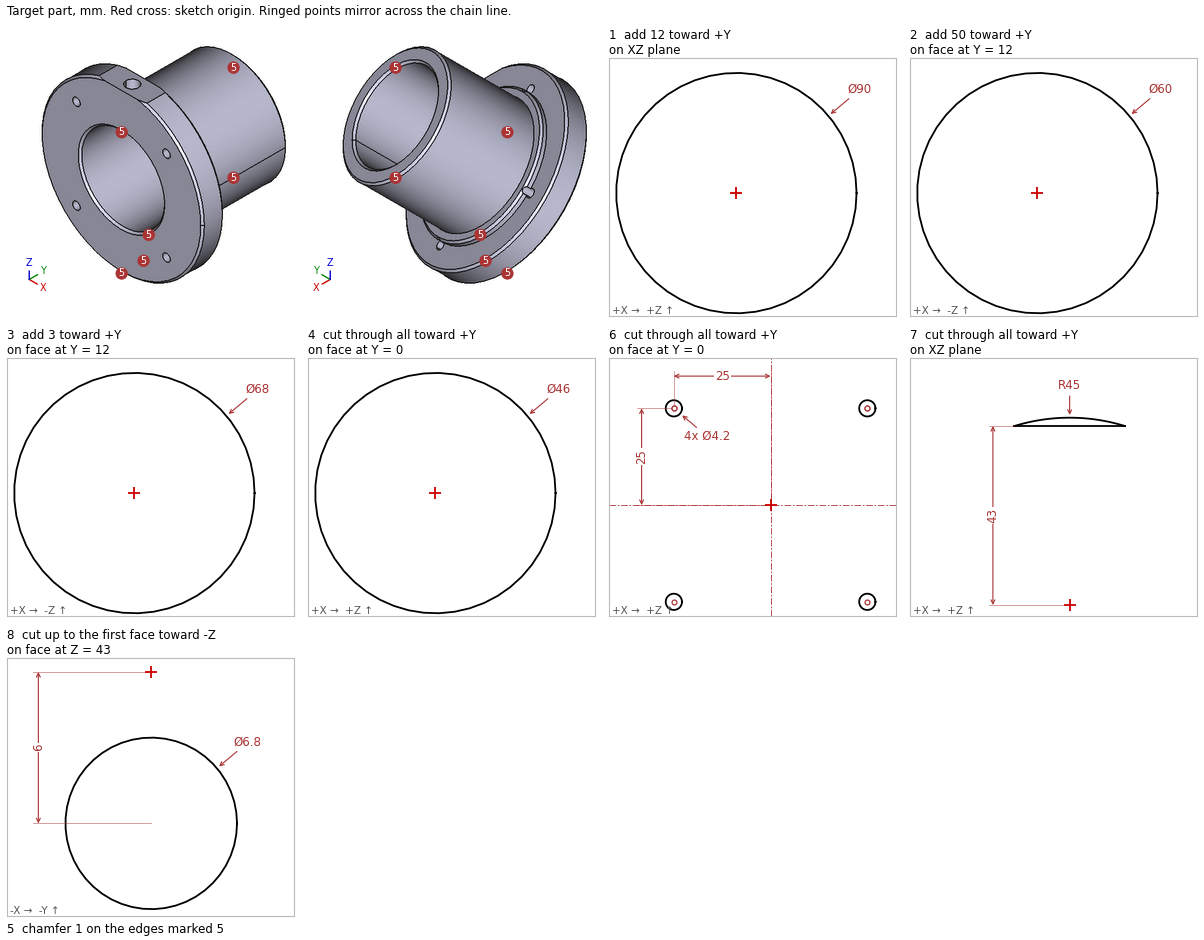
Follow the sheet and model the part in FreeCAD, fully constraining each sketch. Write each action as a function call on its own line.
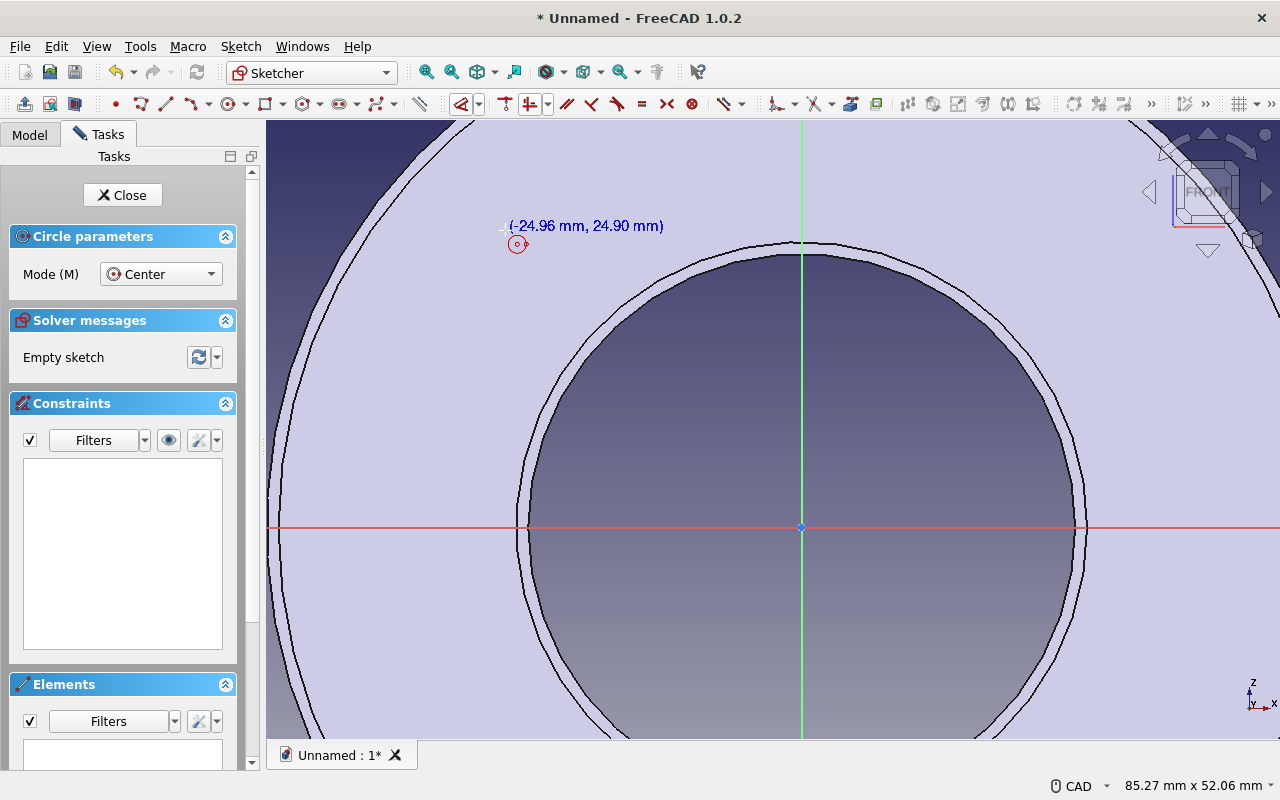
click(504, 230)
move(522, 213)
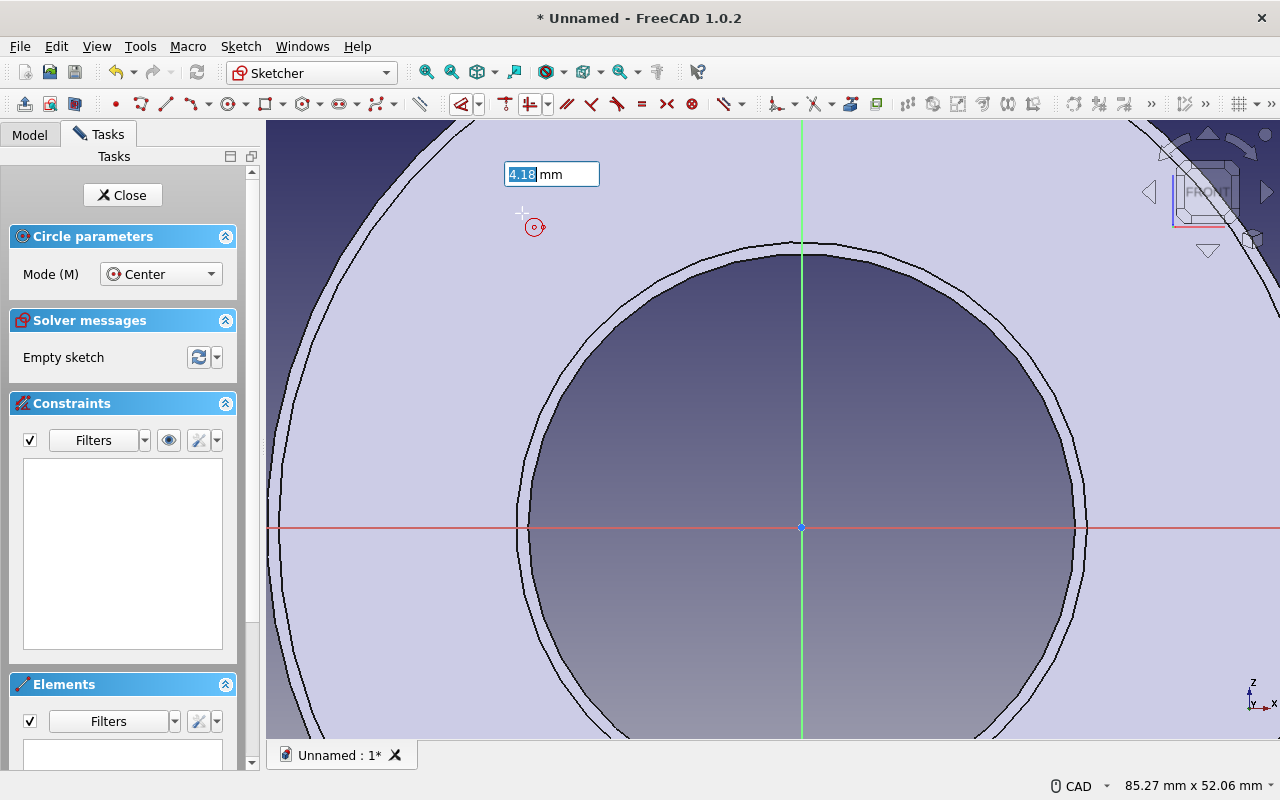
text(4.2)
key(Return)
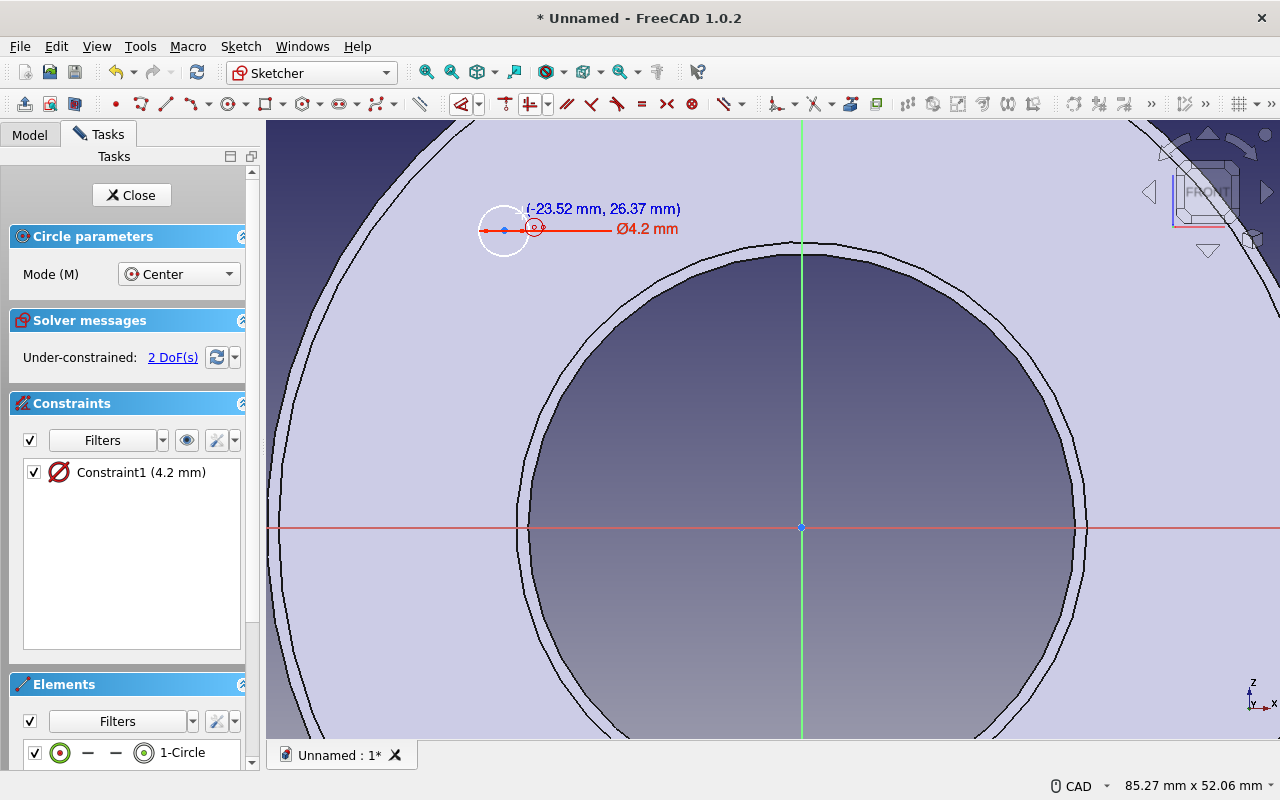
click(1099, 230)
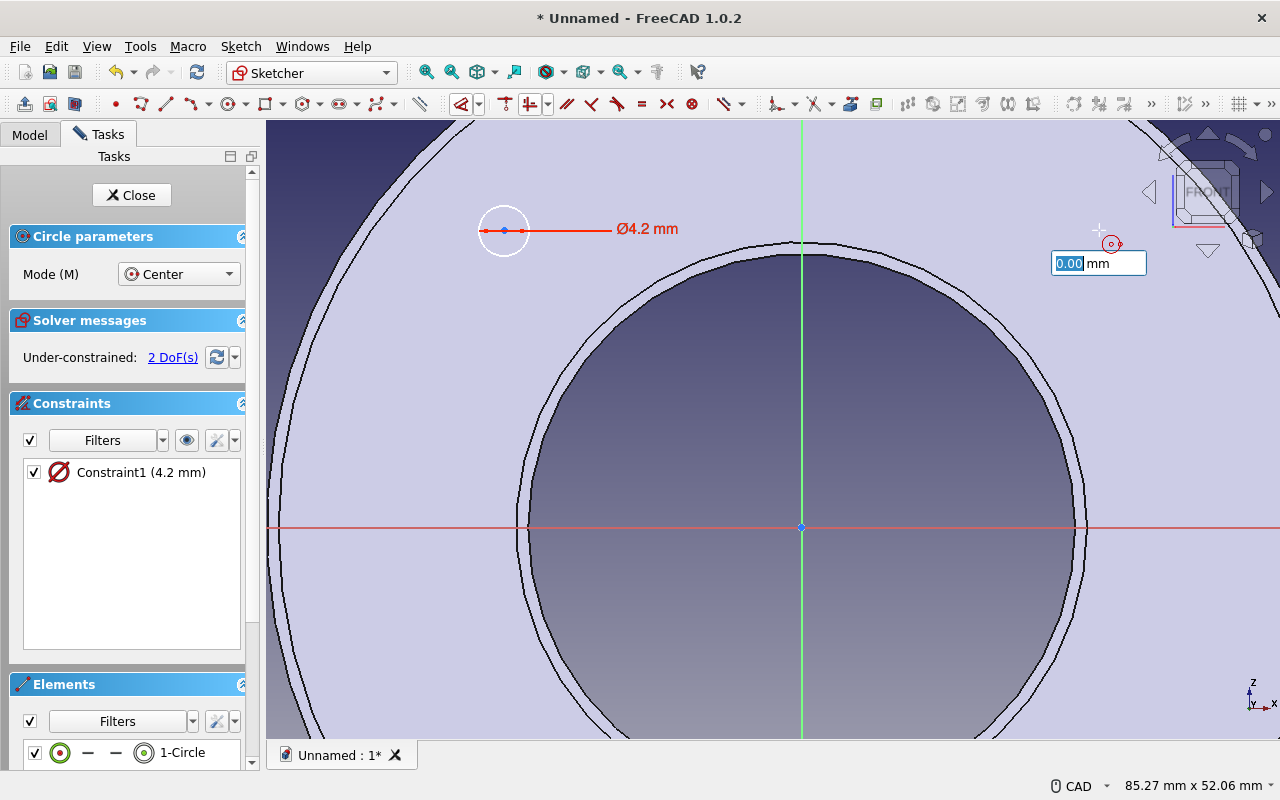
scroll(507, 230, down, 2)
move(916, 218)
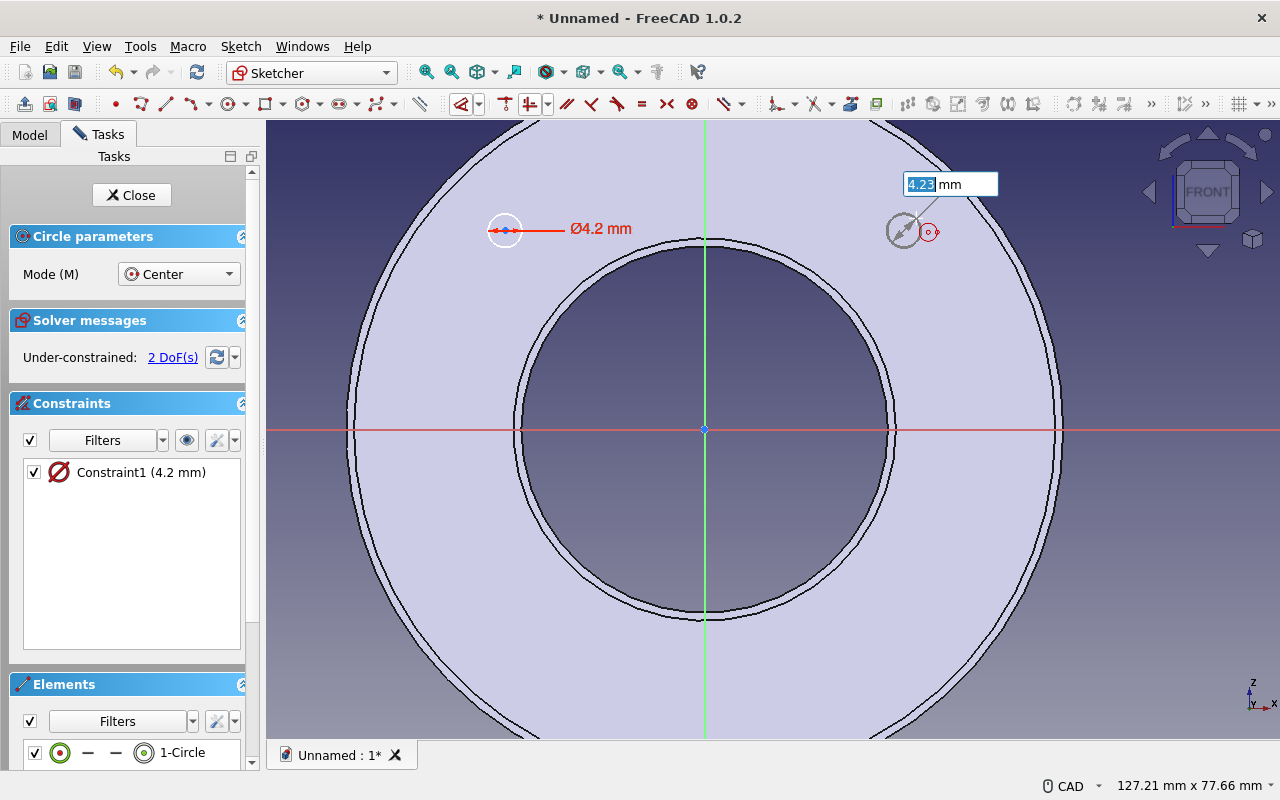
text(4.2)
key(Return)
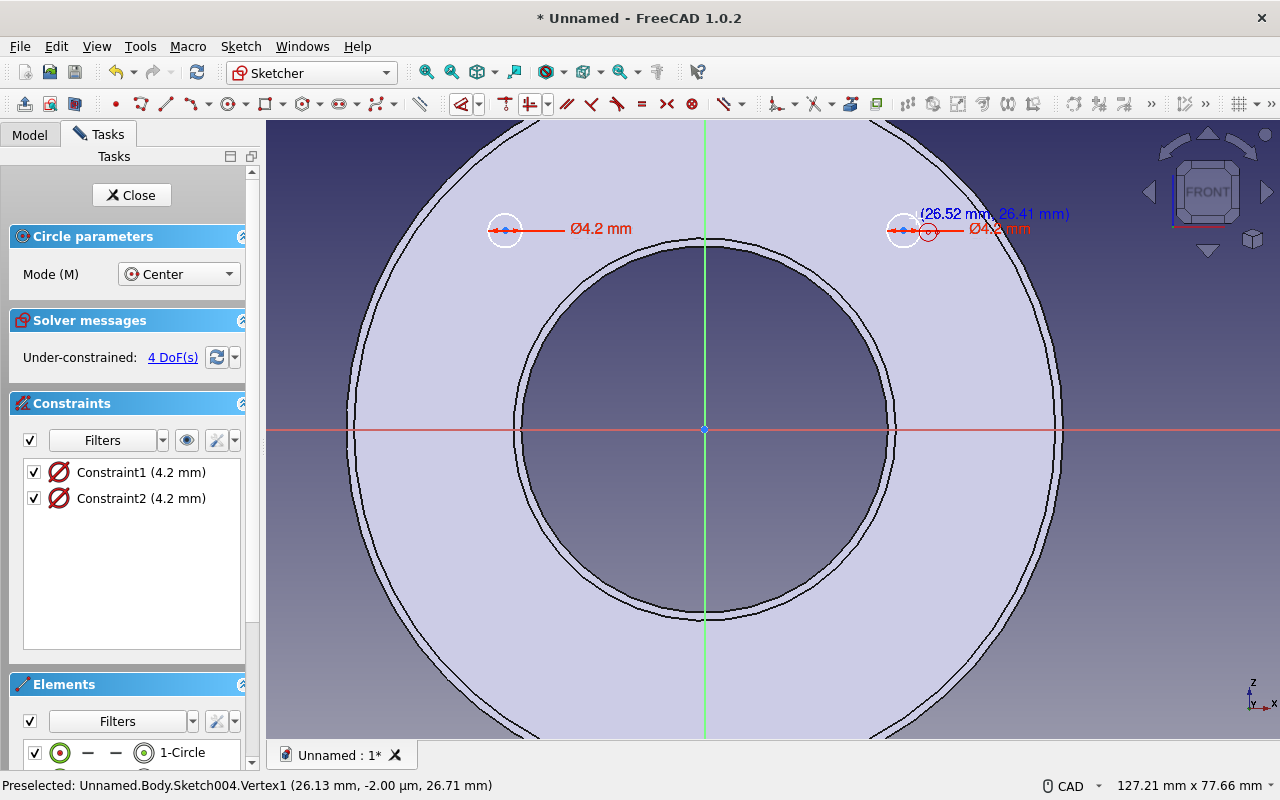
scroll(904, 629, up, 2)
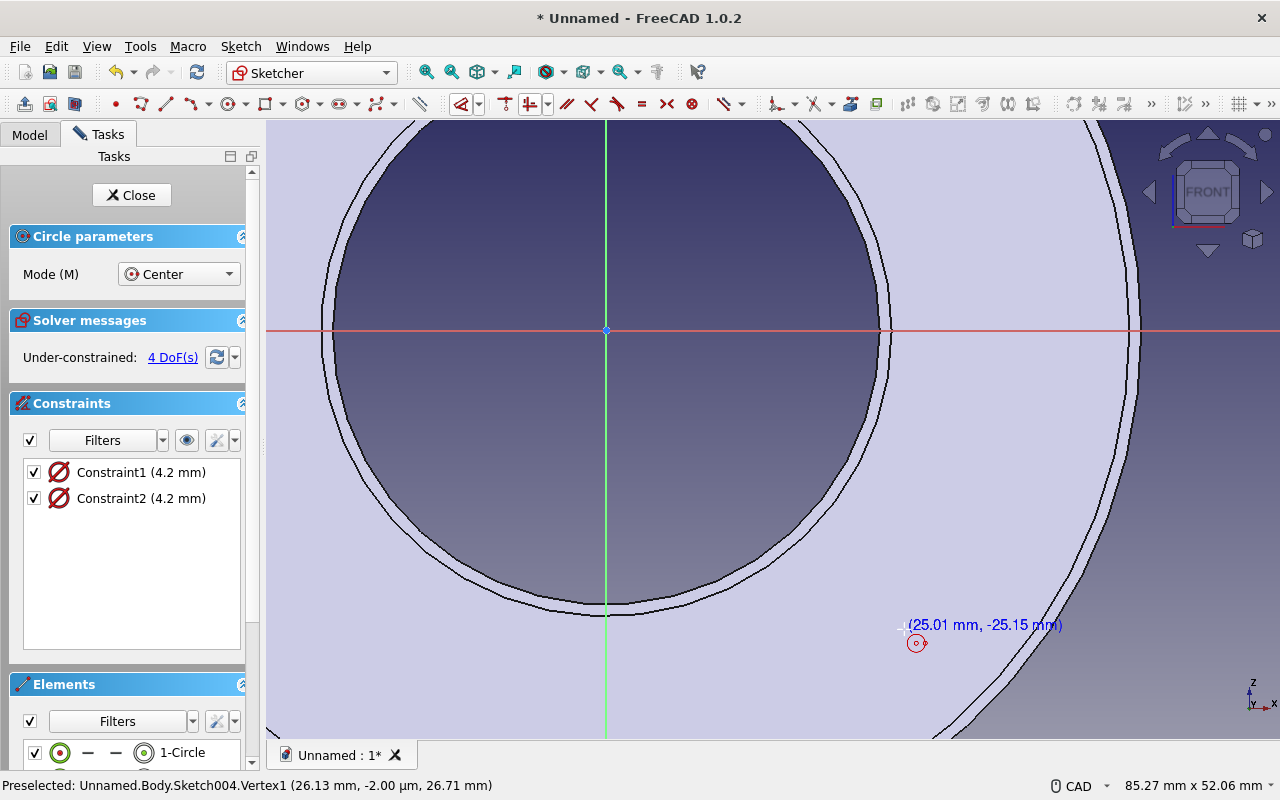
click(904, 628)
move(921, 611)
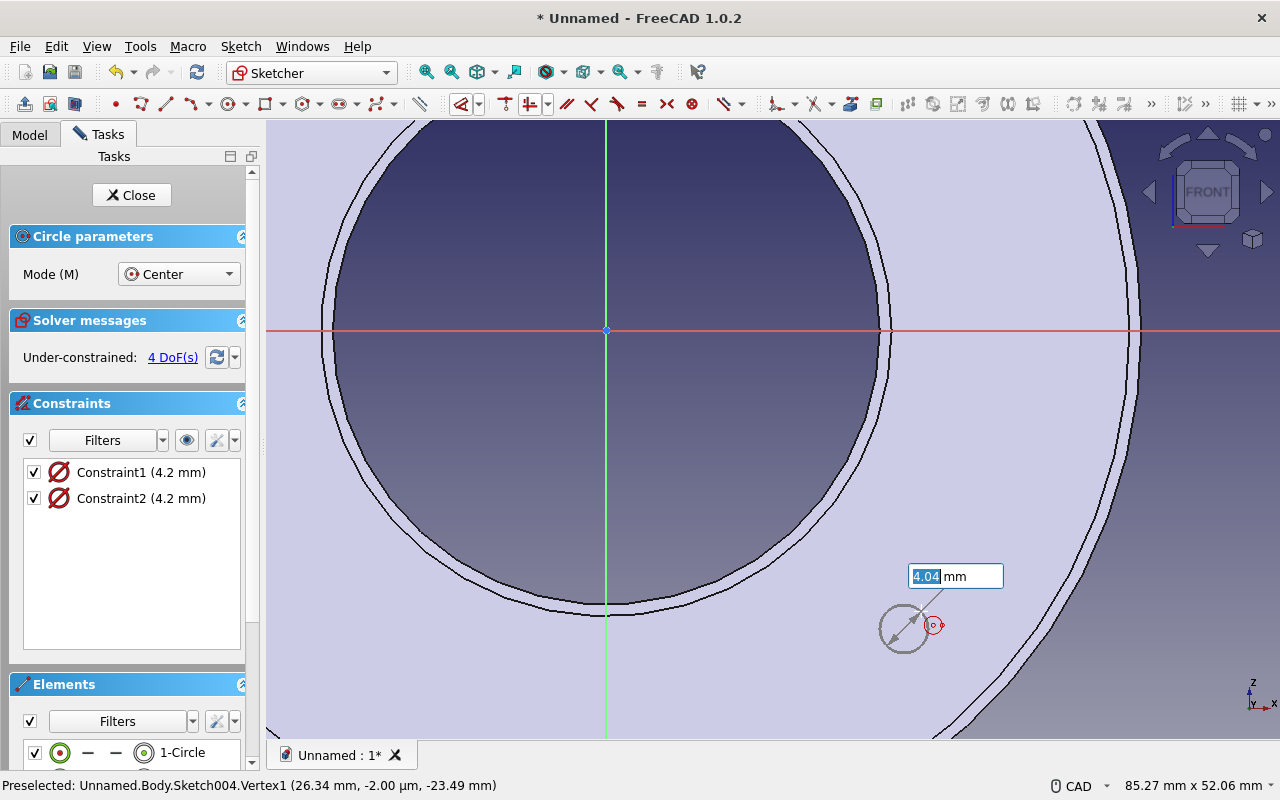
text(4.2)
key(Return)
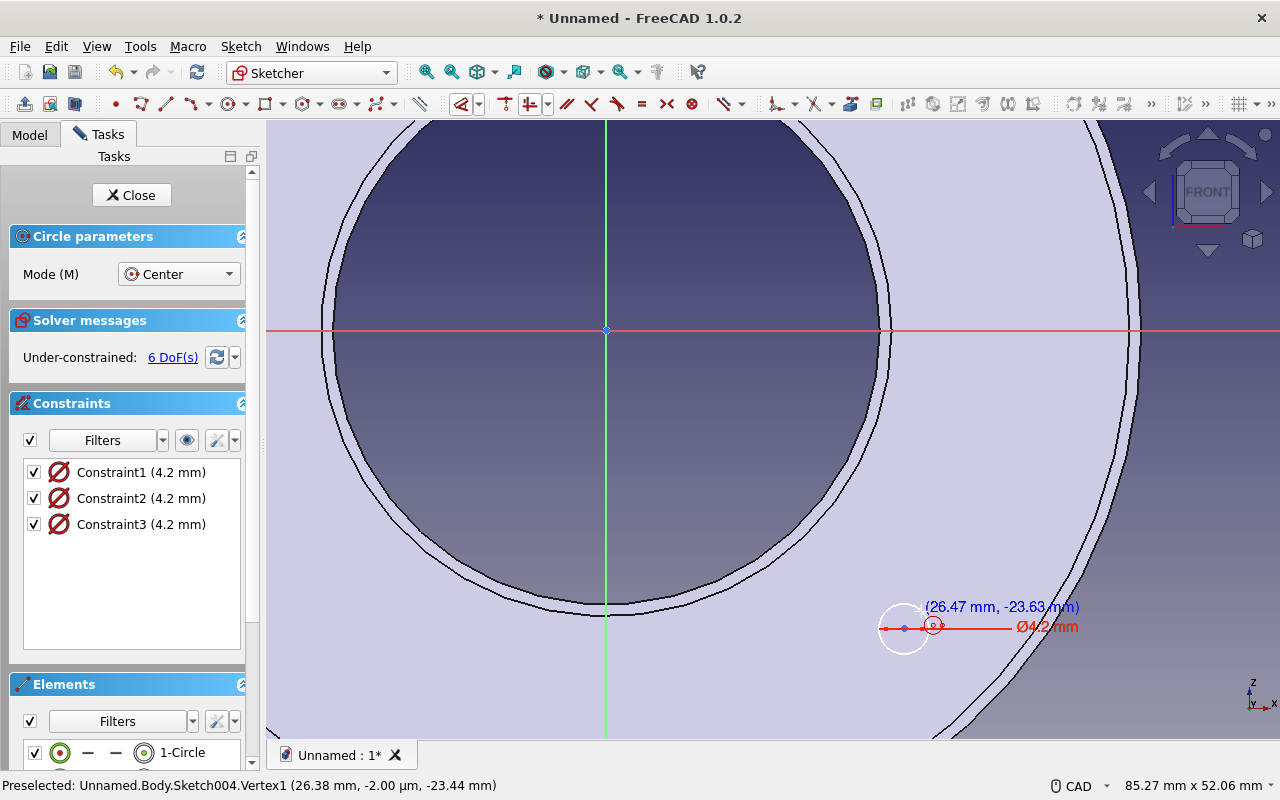
click(309, 628)
move(327, 611)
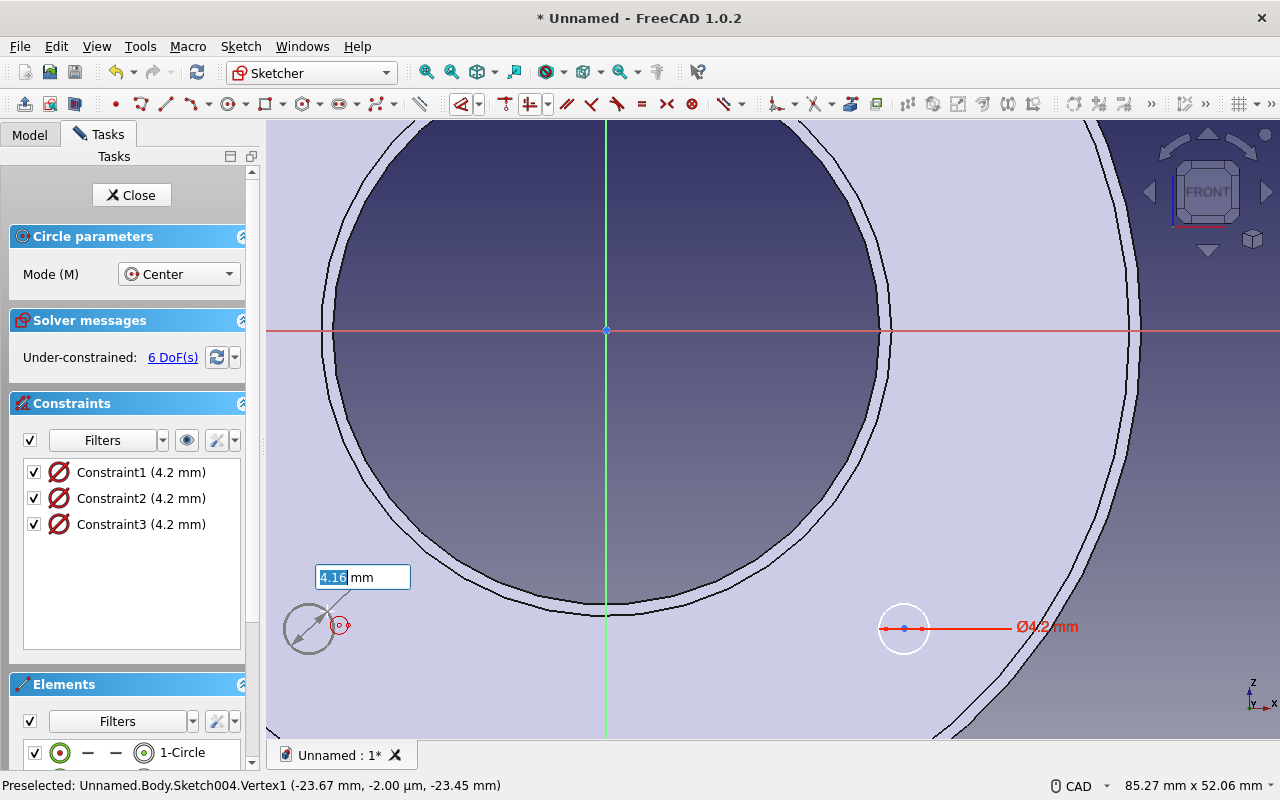
text(4.2)
key(Return)
key(Escape)